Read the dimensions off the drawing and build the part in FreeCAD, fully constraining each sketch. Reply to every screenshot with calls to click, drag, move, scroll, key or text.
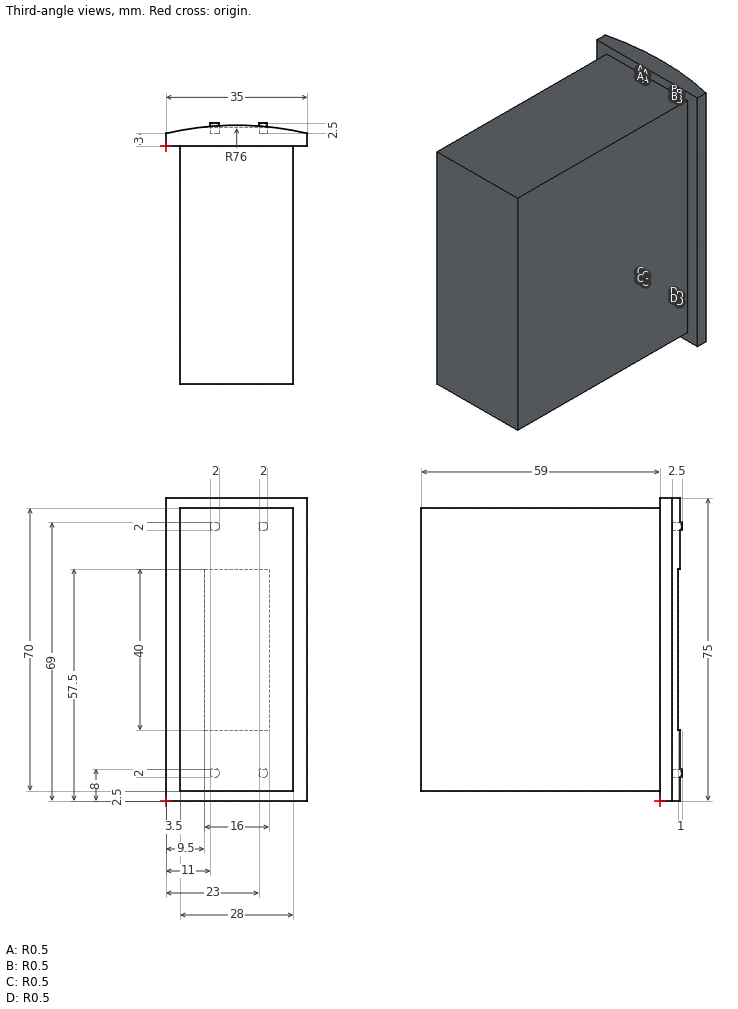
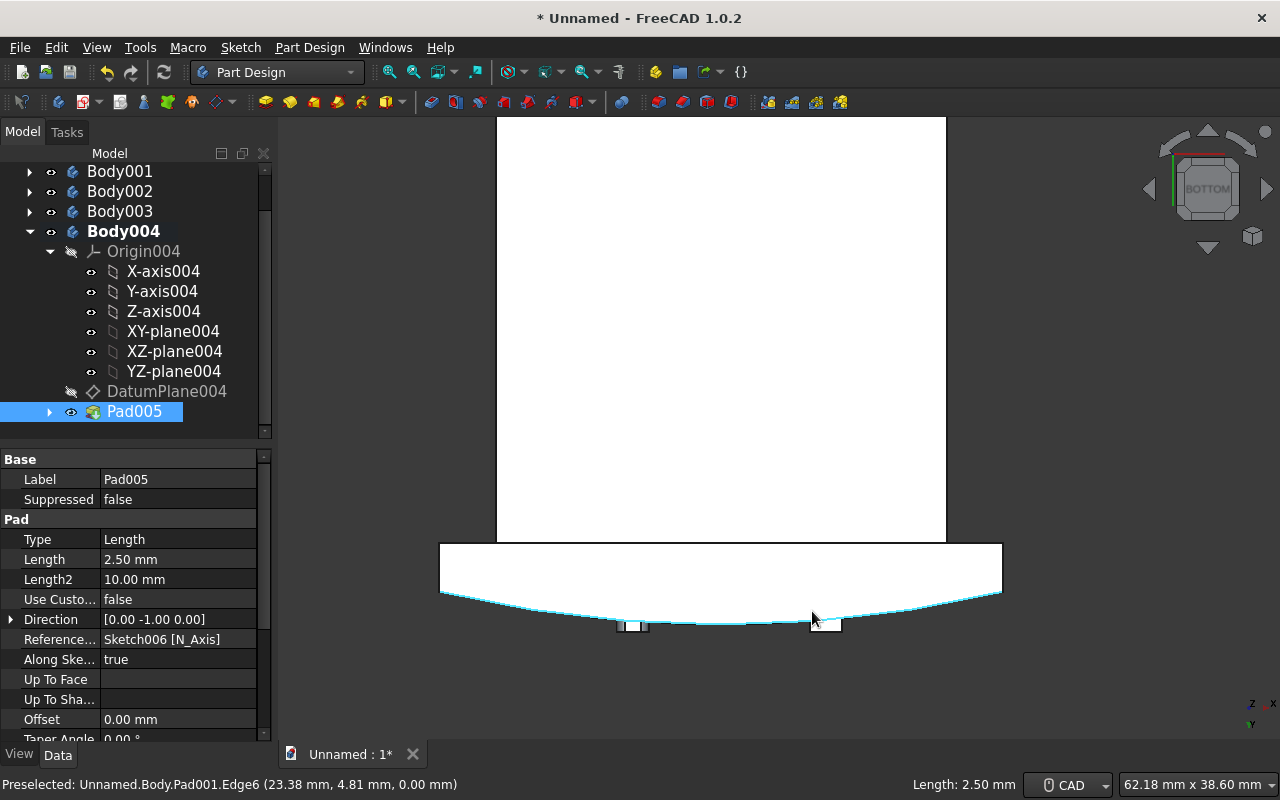
click(842, 623, ctrl)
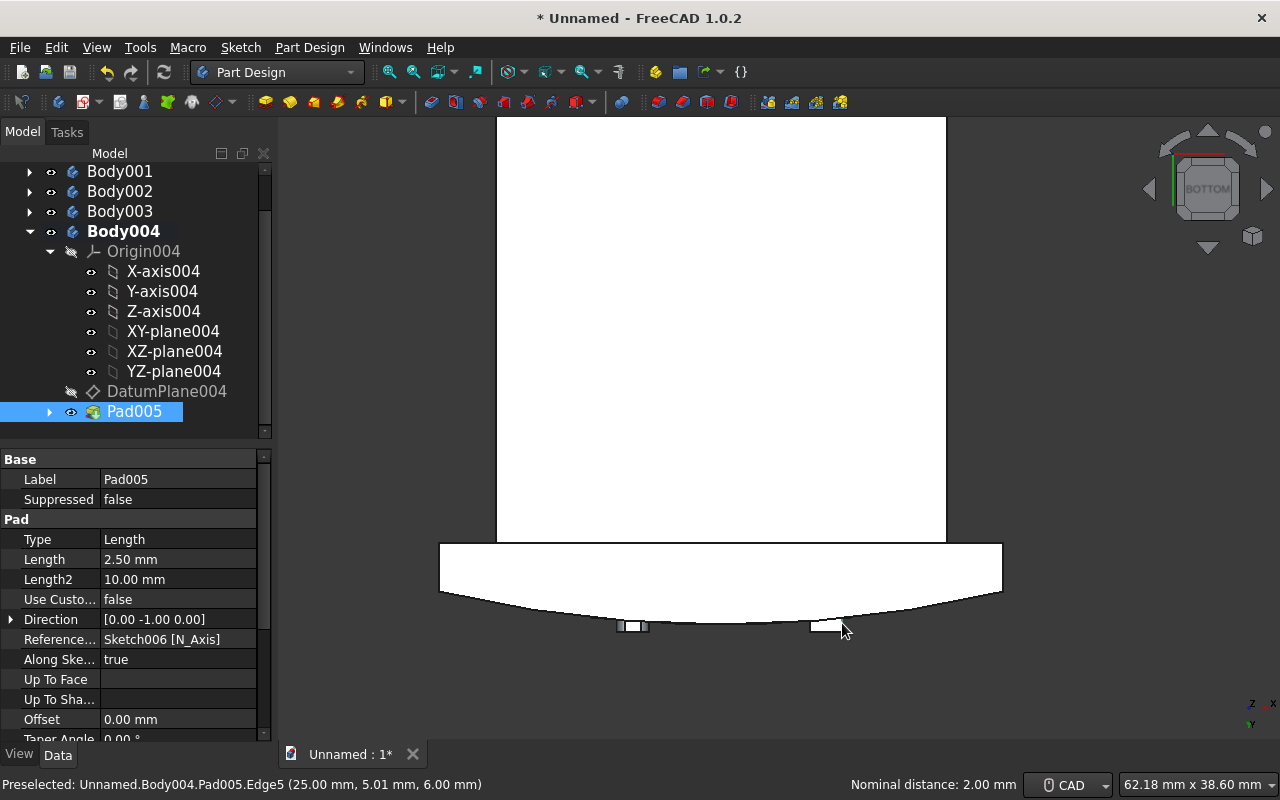
key(v)
key(f)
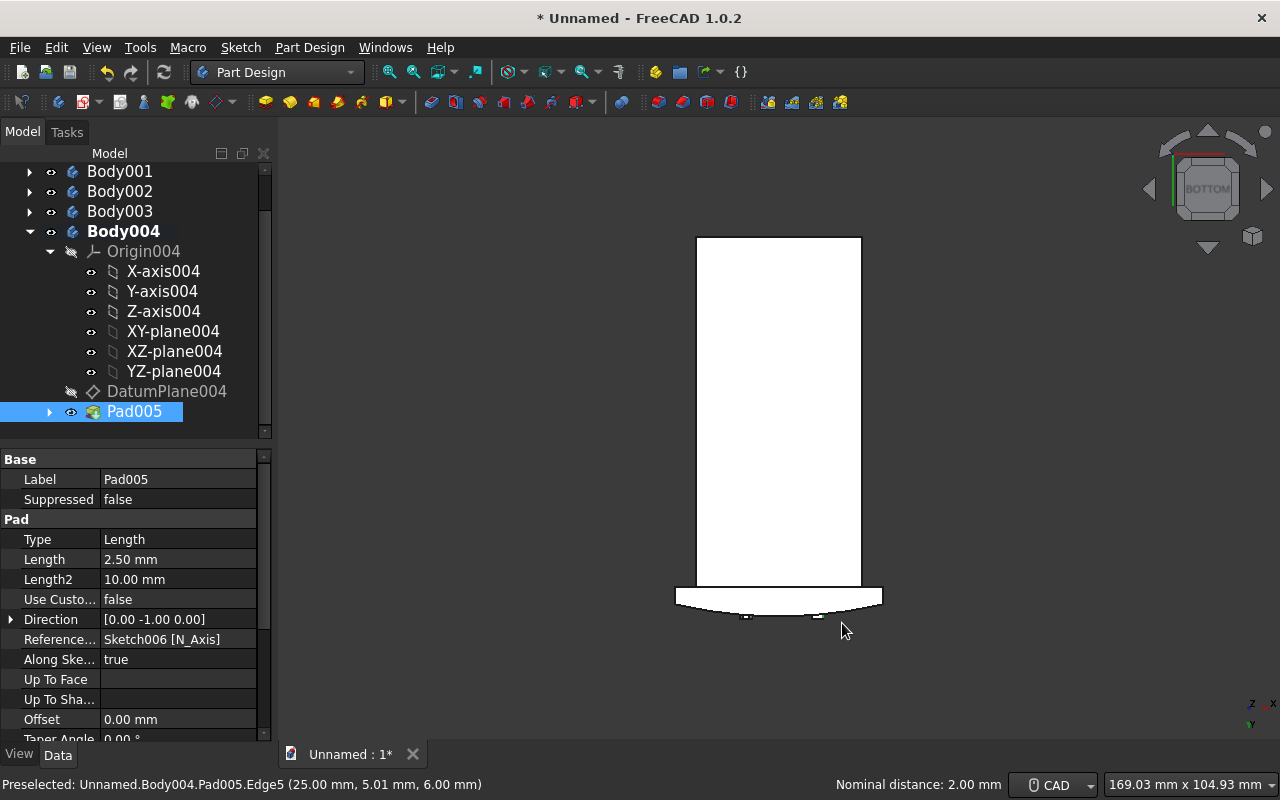
key(4)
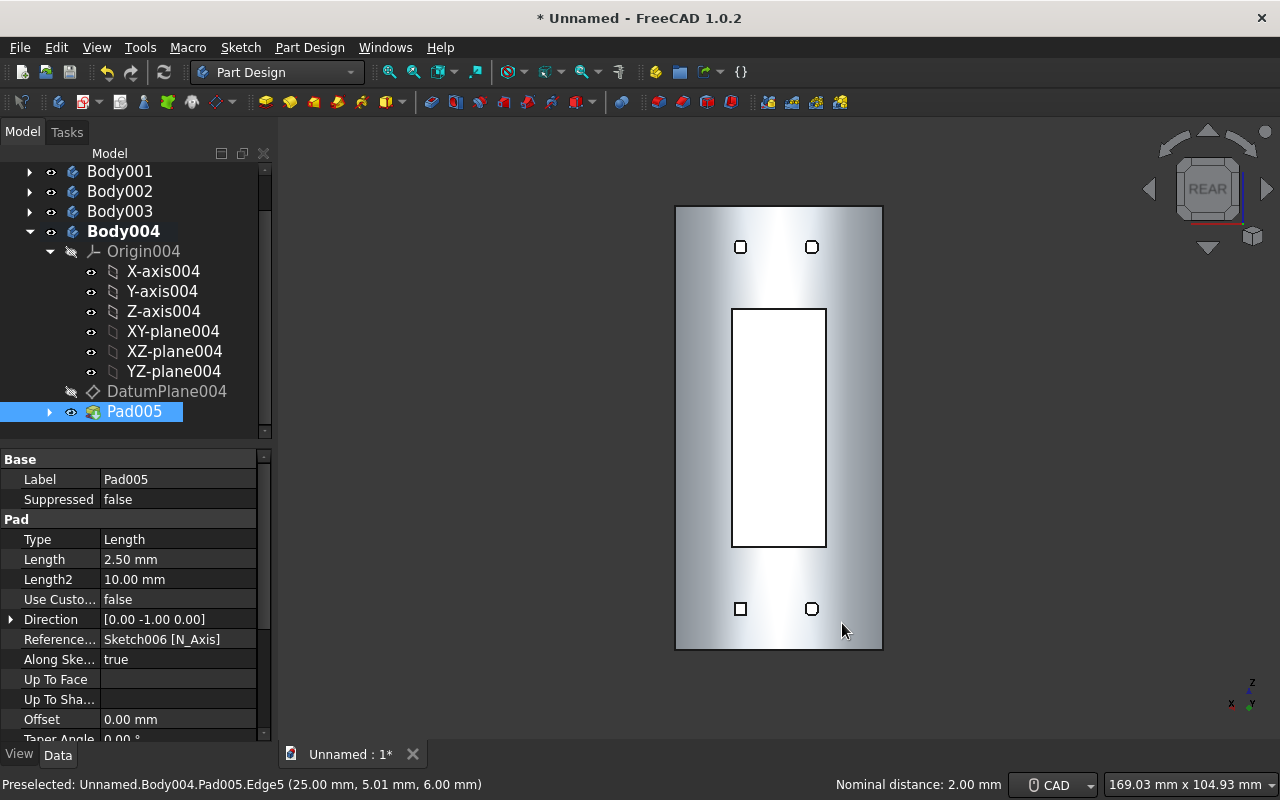
key(v)
key(f)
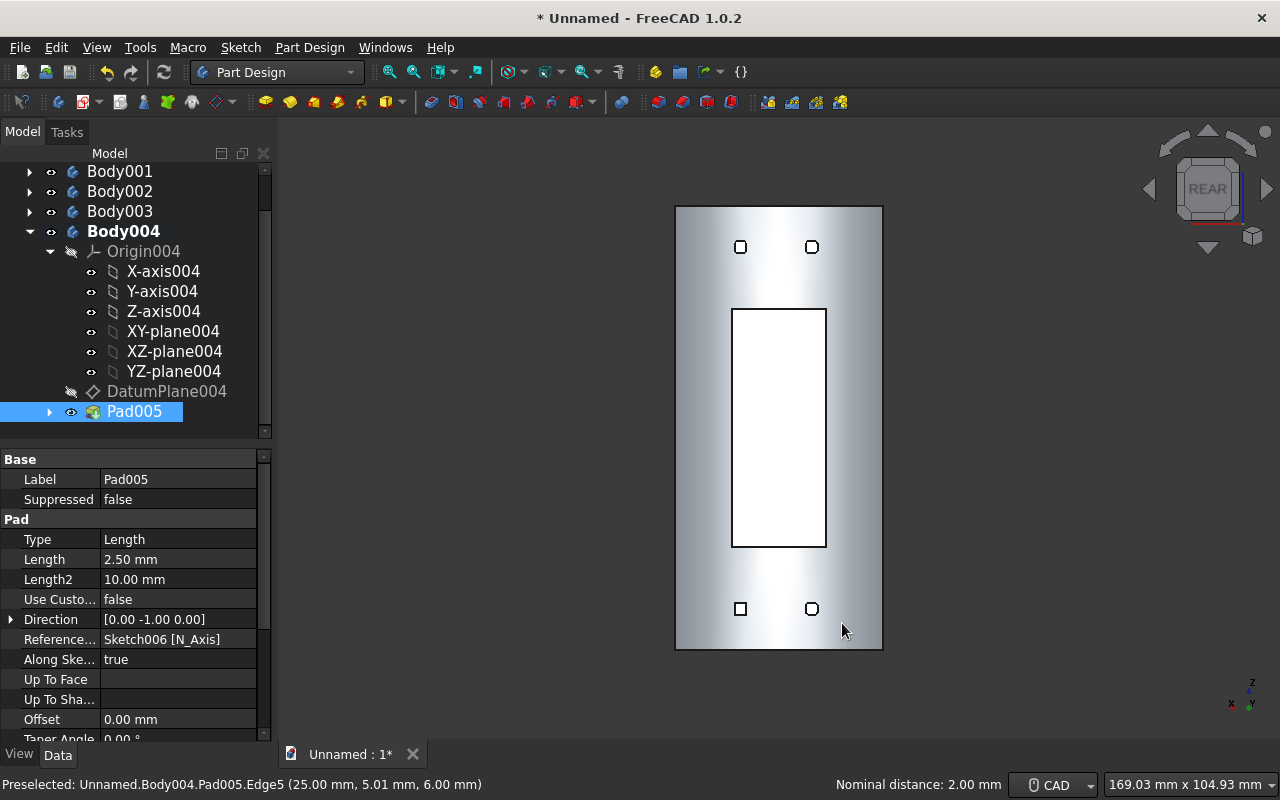
scroll(746, 602, up, 5)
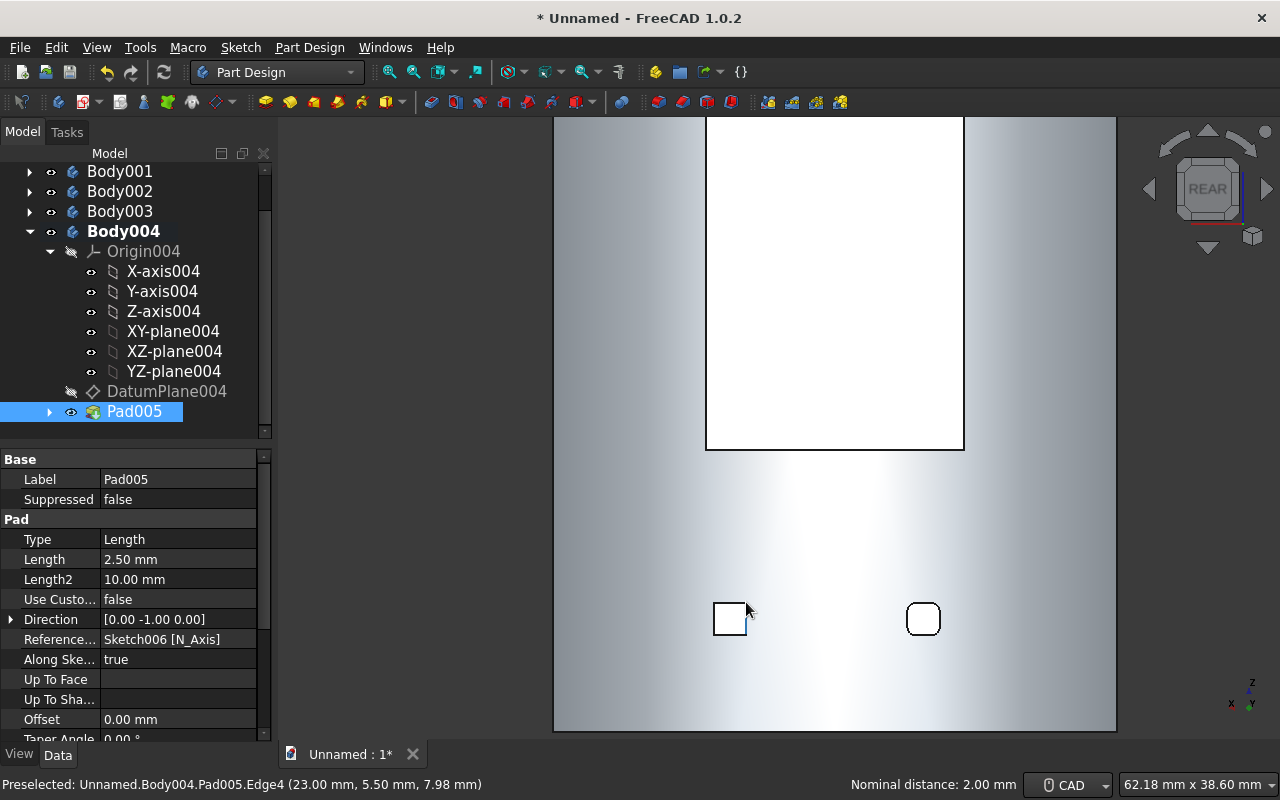
key(v)
key(f)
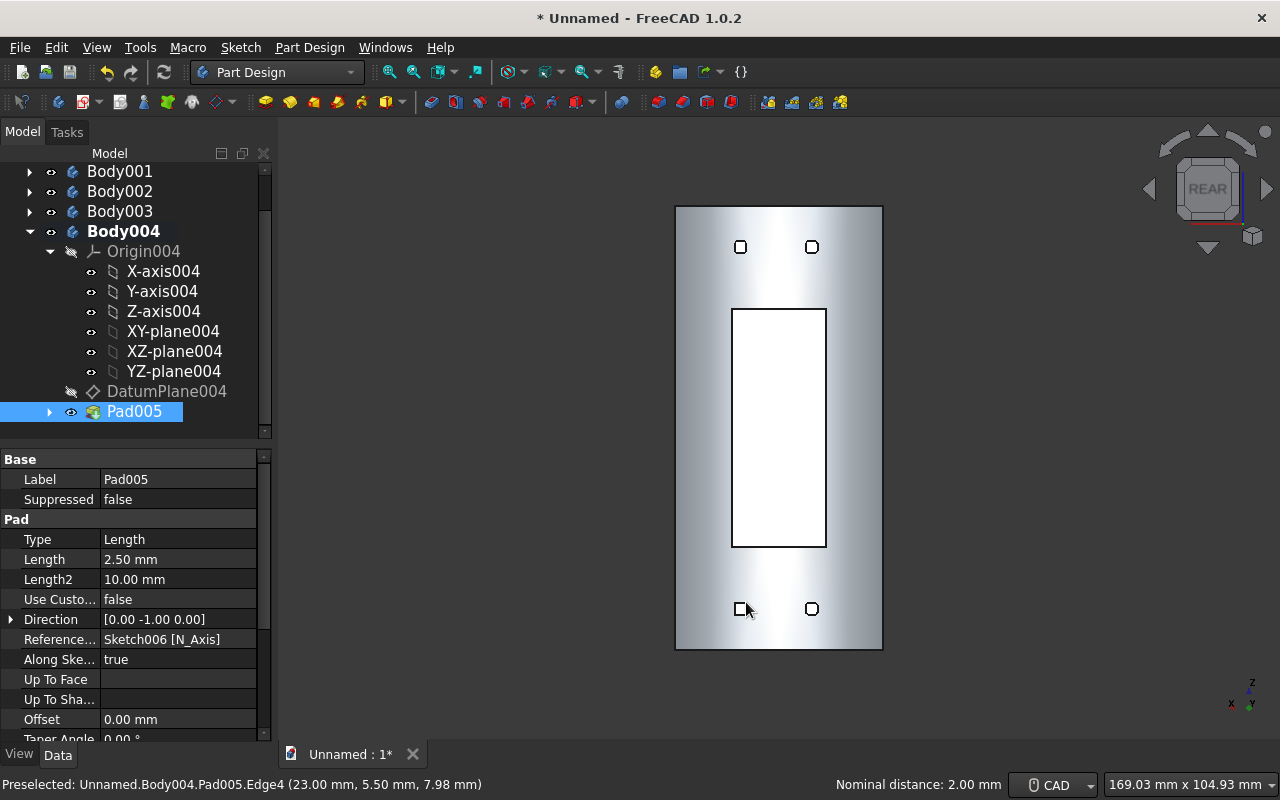
key(6)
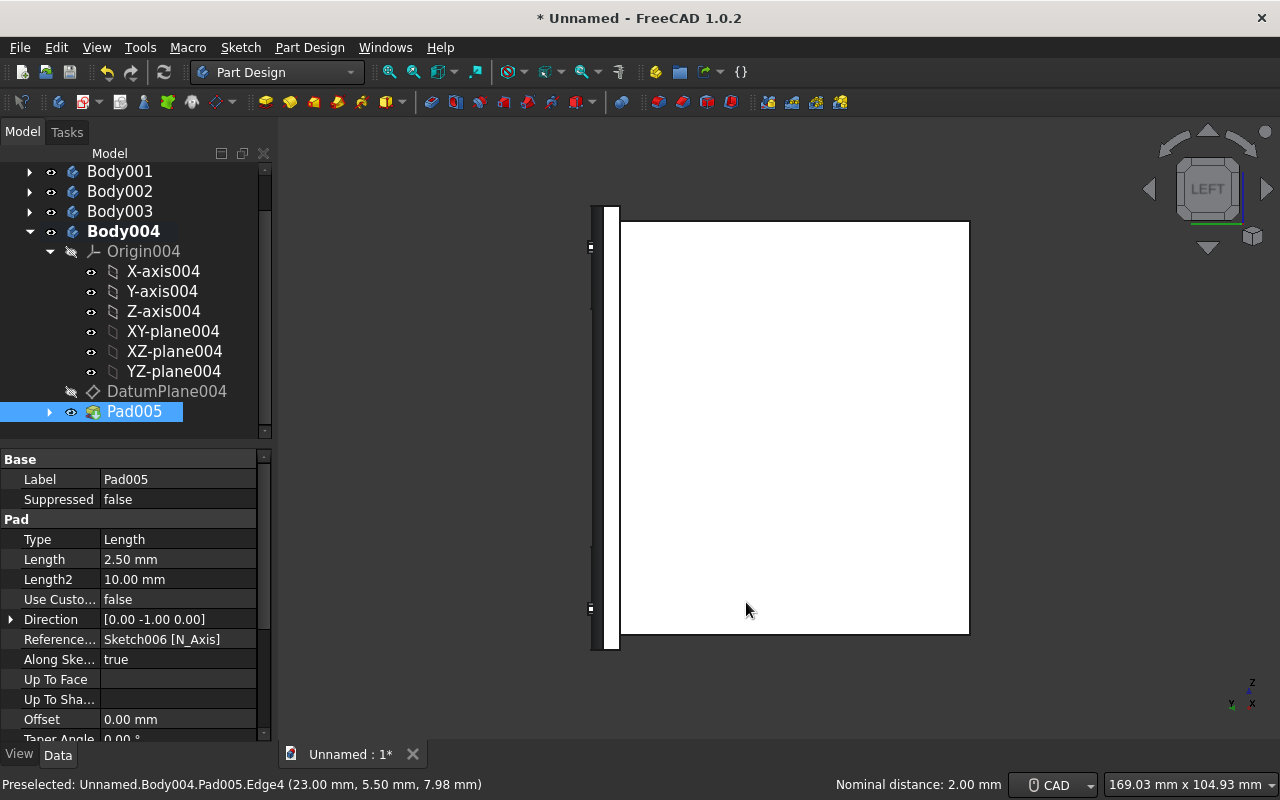
key(v)
key(f)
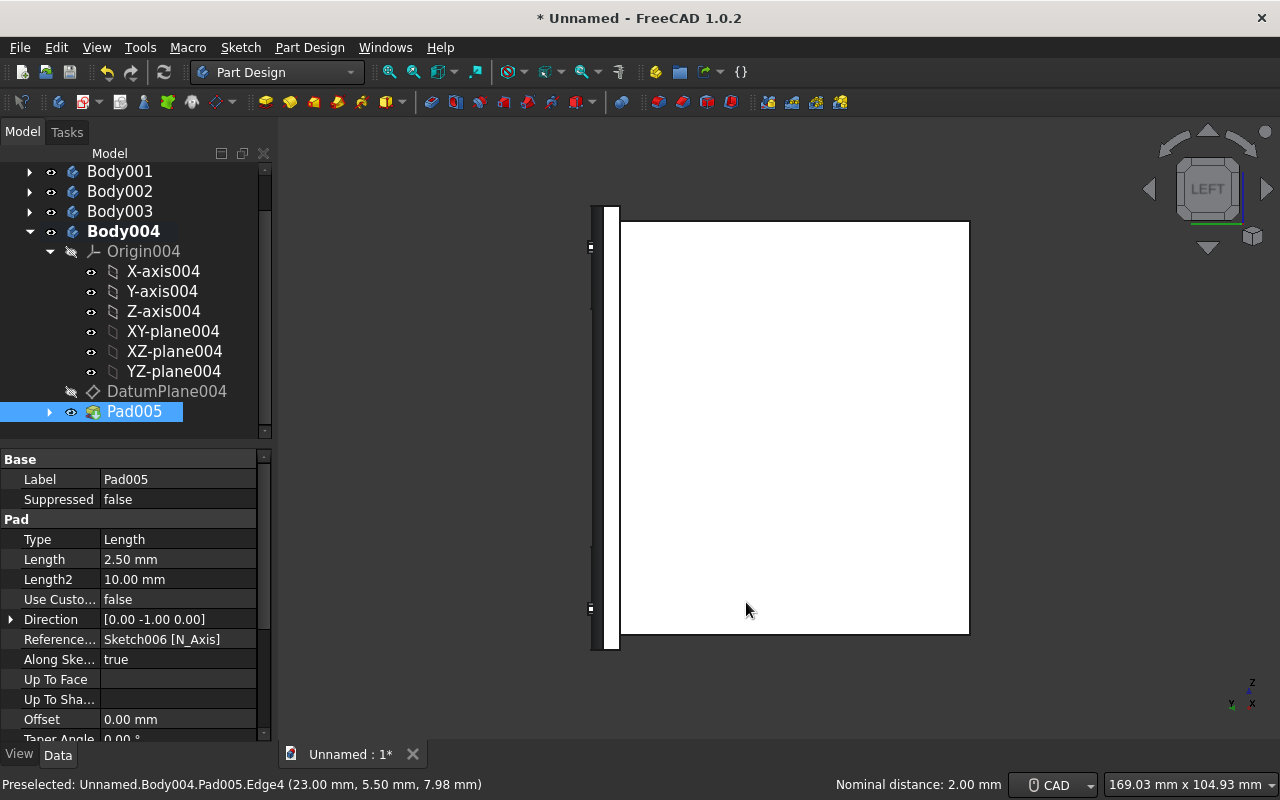
scroll(595, 602, up, 5)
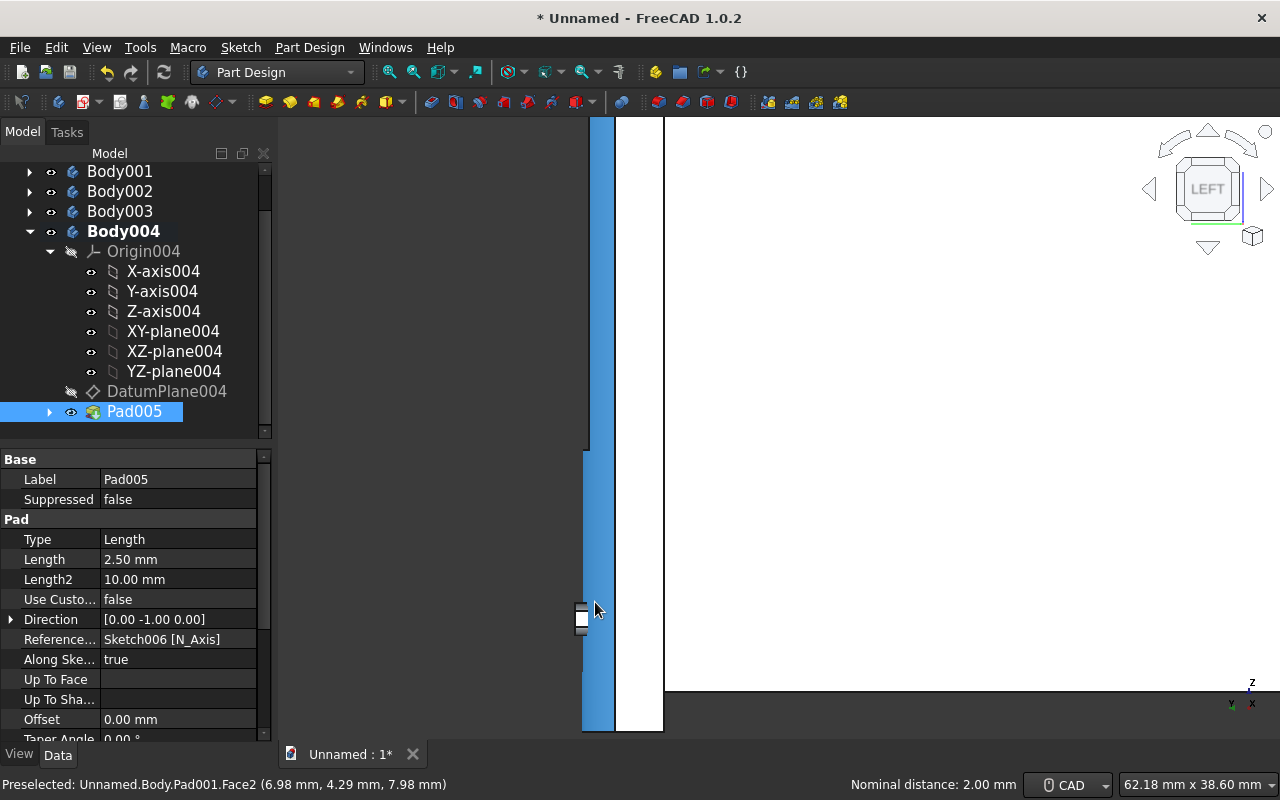
key(v)
key(f)